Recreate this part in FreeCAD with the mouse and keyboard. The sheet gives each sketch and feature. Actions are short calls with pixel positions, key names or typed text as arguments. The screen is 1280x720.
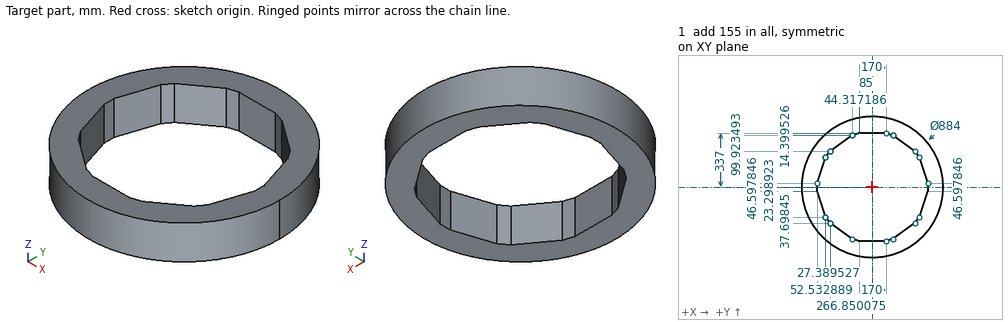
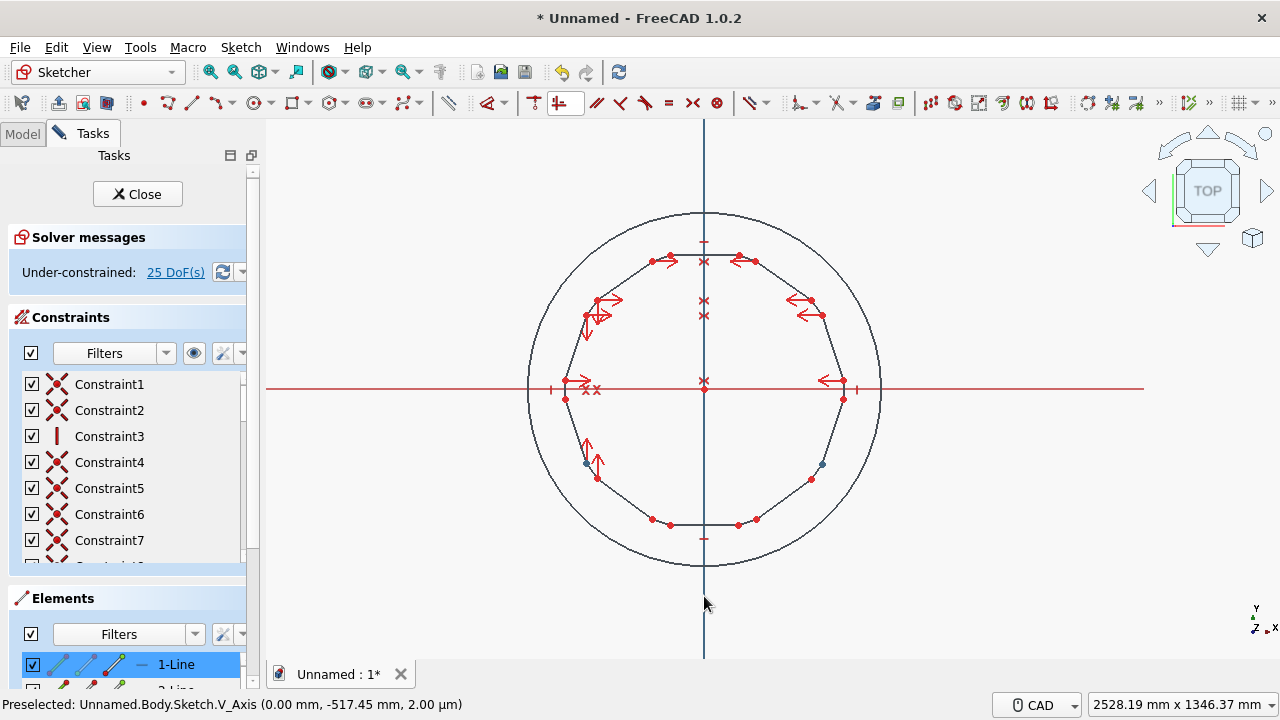
key(s)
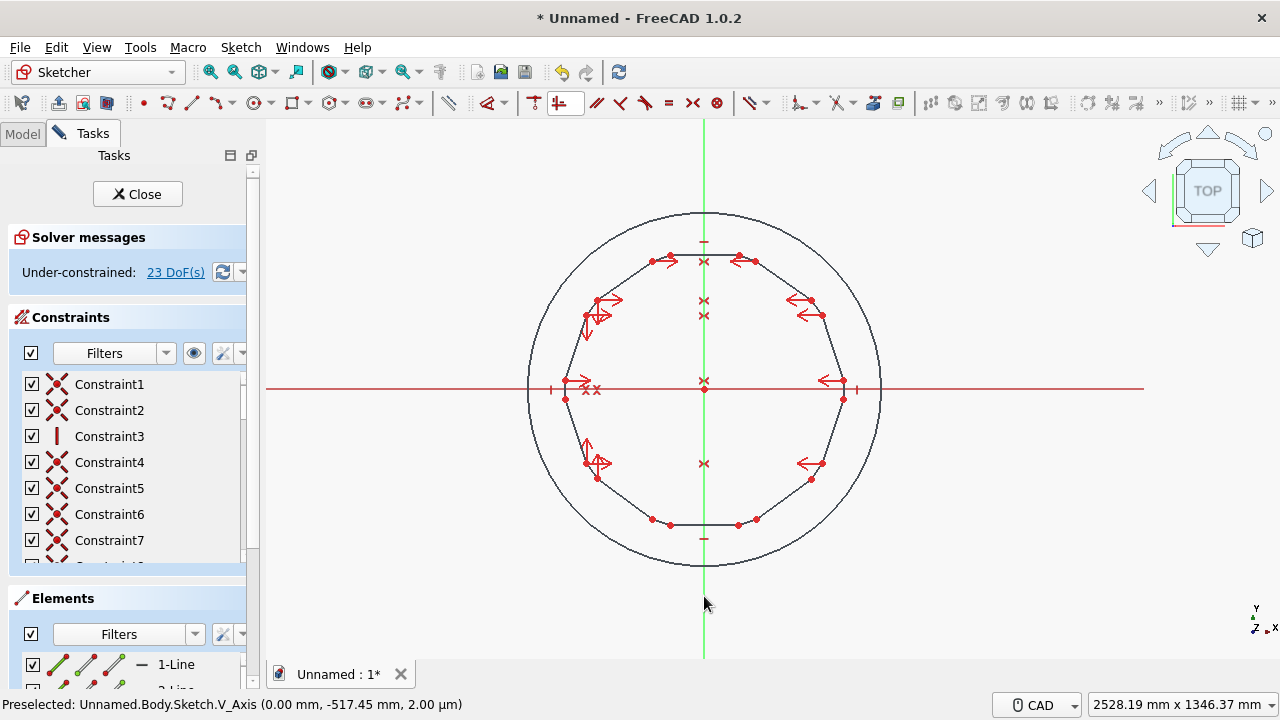
click(598, 479)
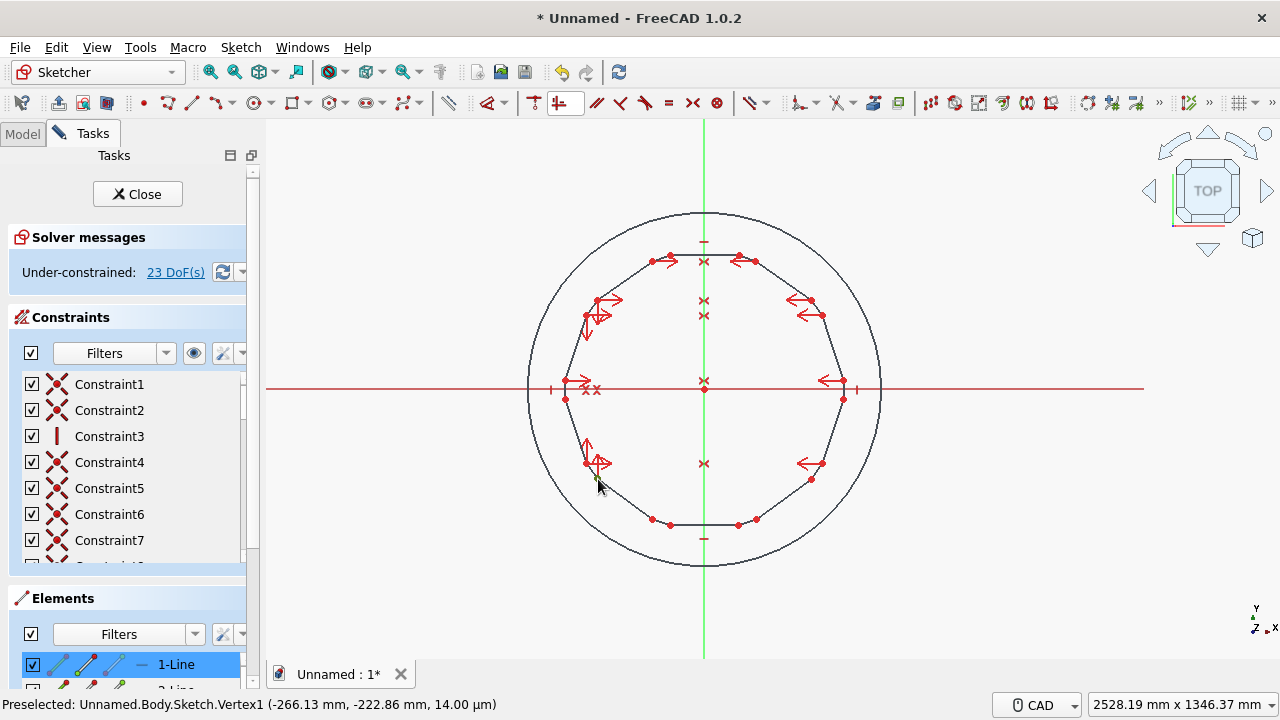
click(811, 479)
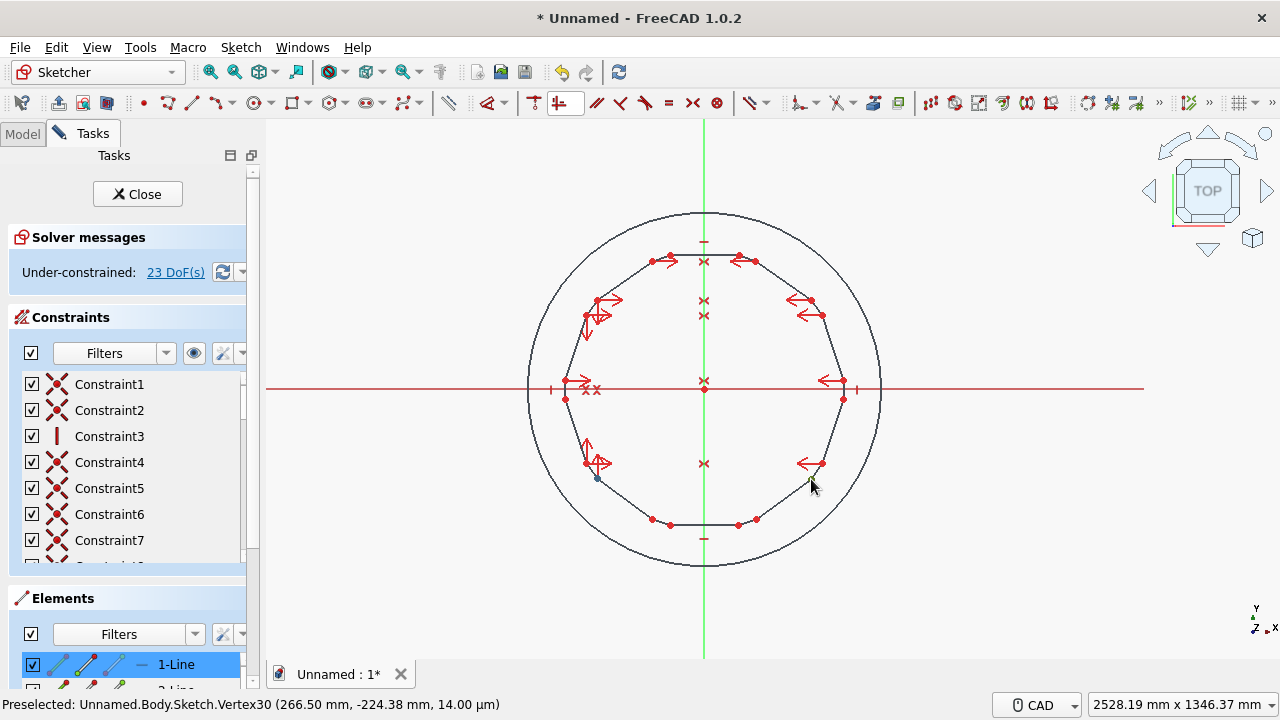
click(704, 596)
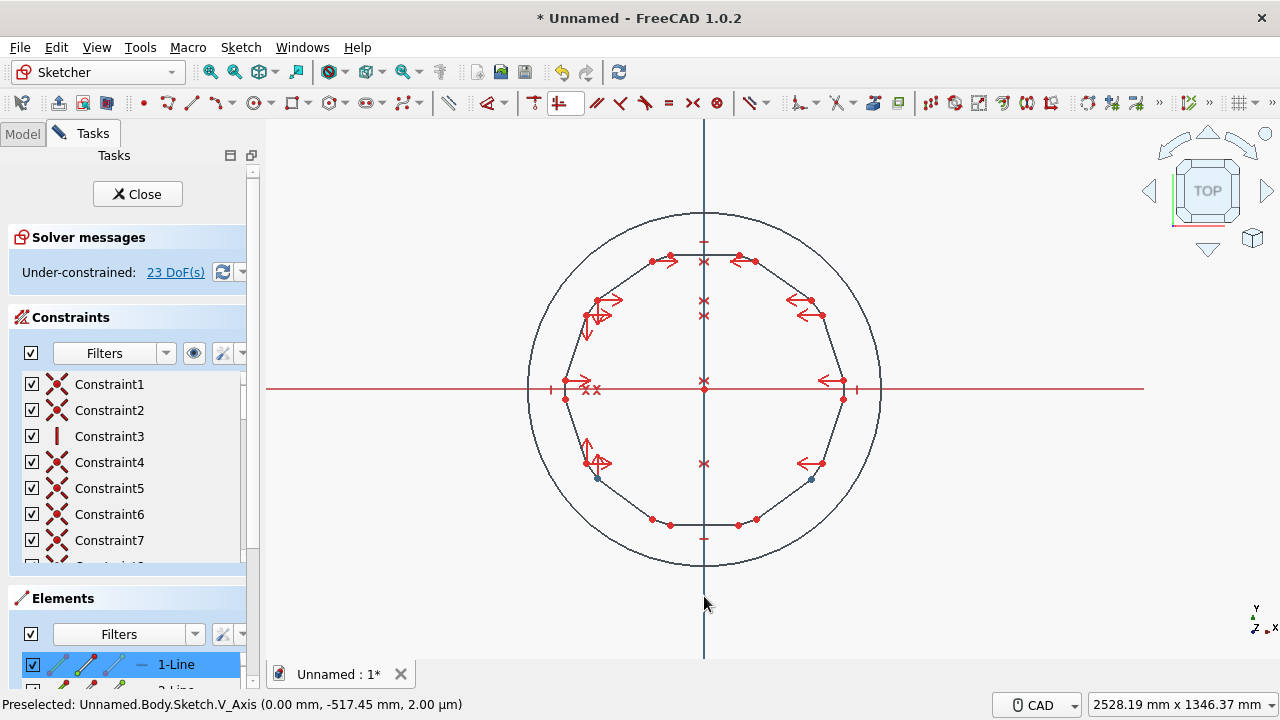
click(694, 104)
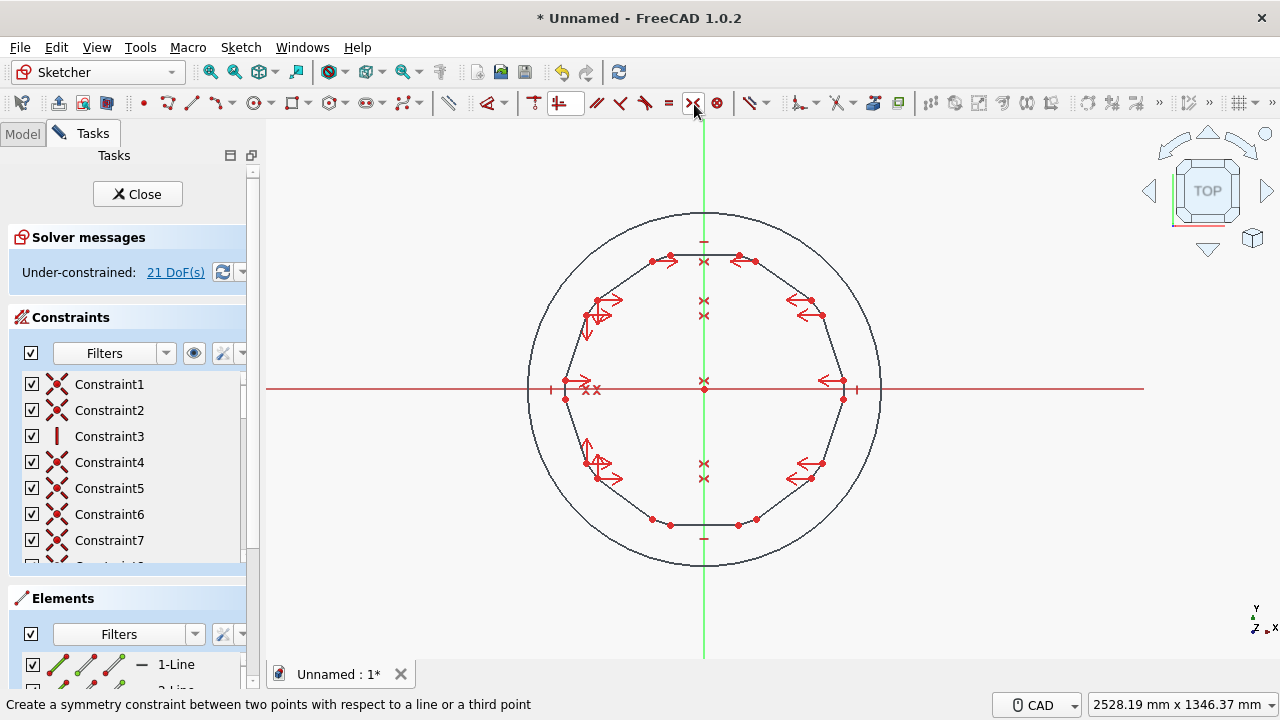
click(756, 261)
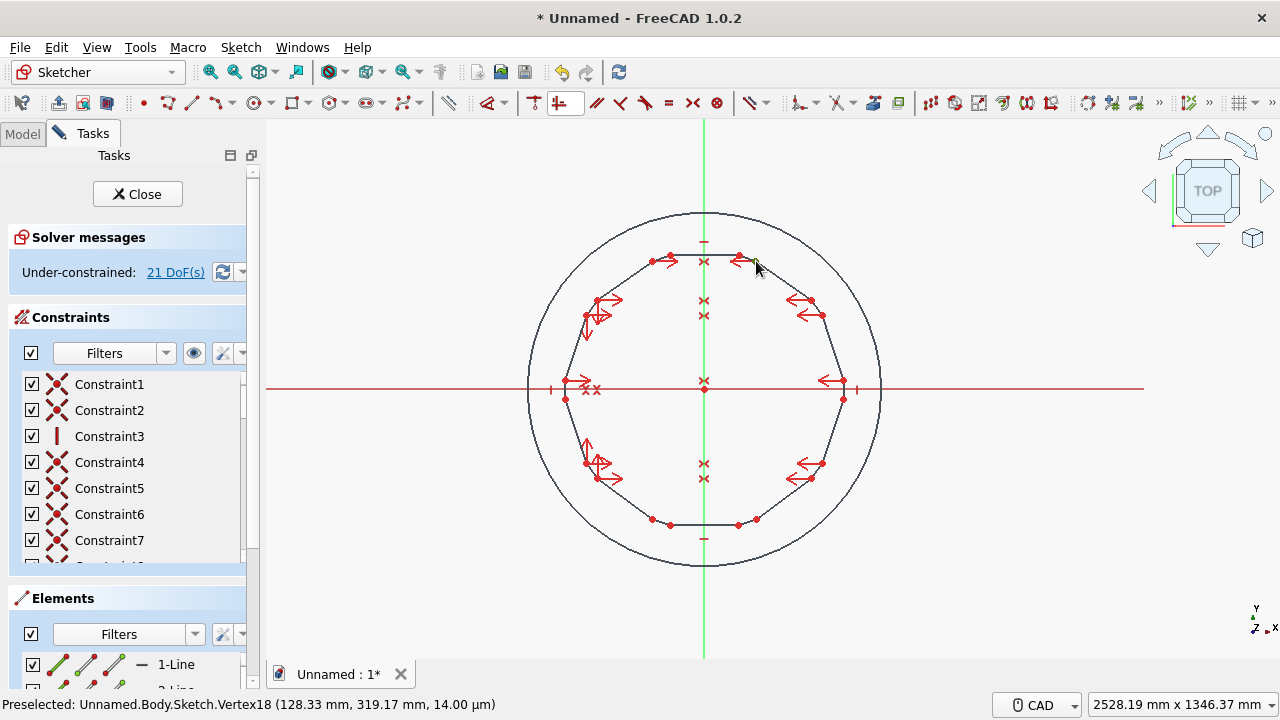
click(757, 519)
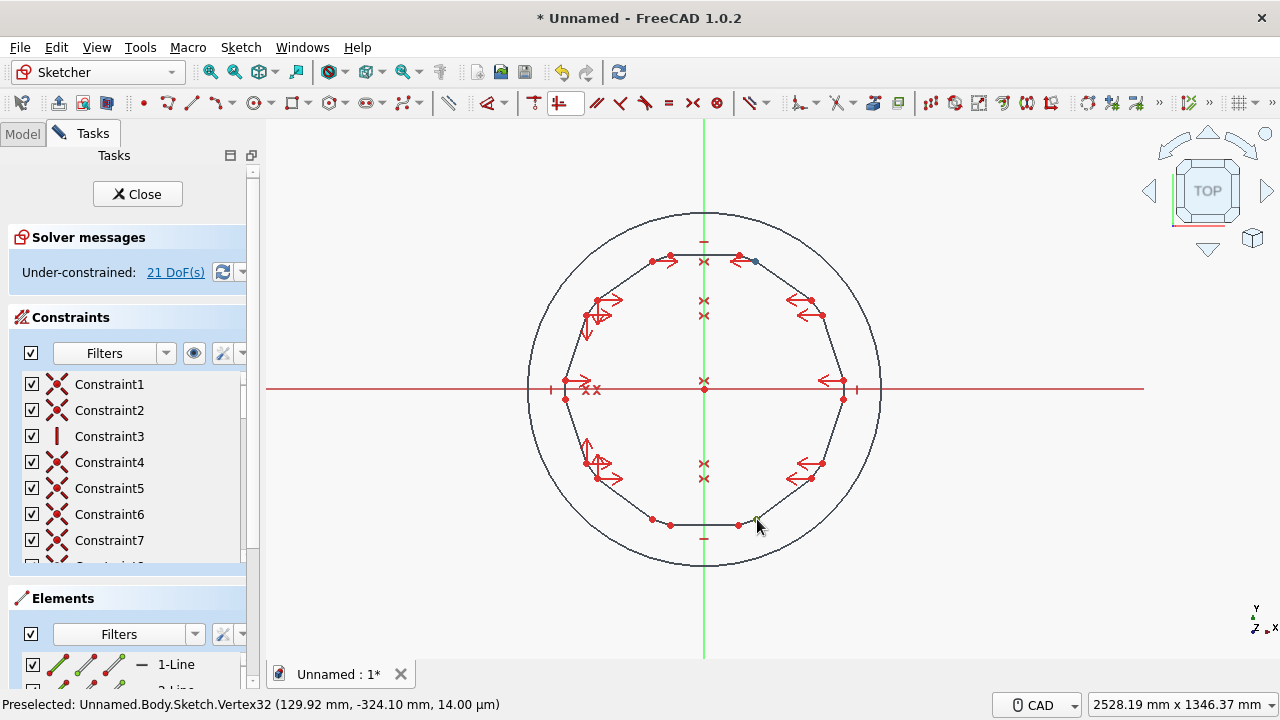
click(353, 389)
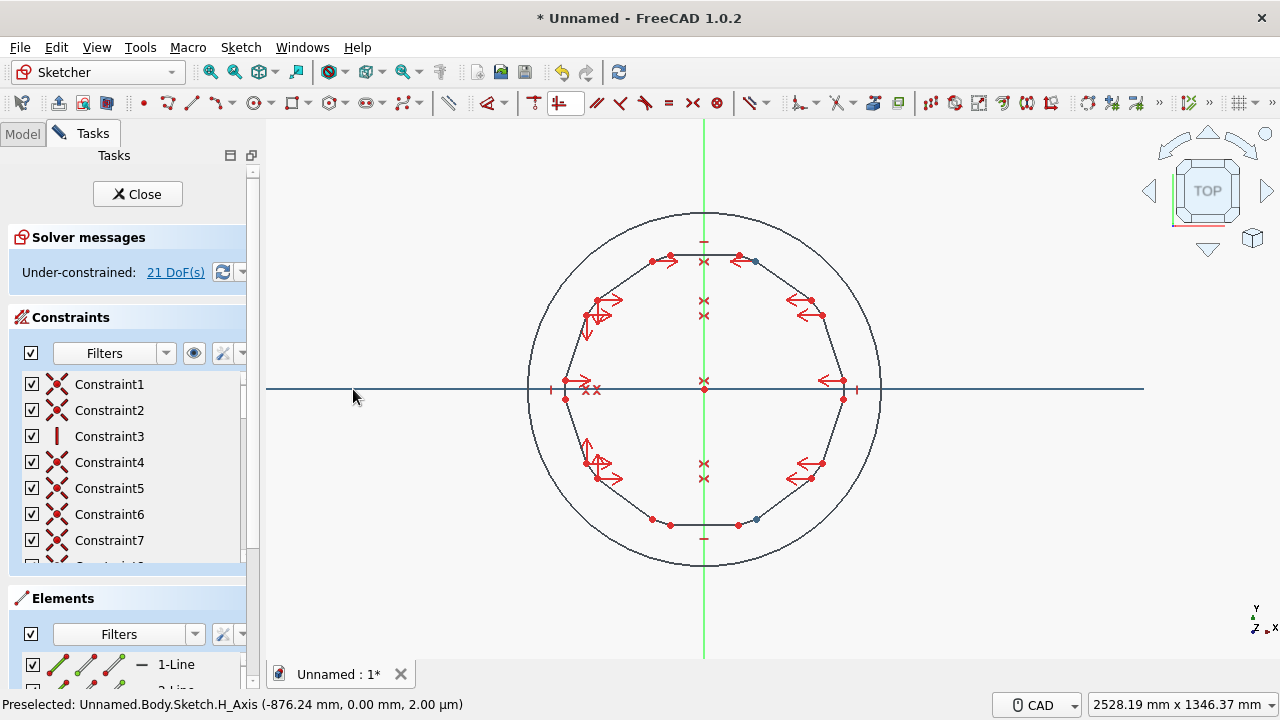
key(s)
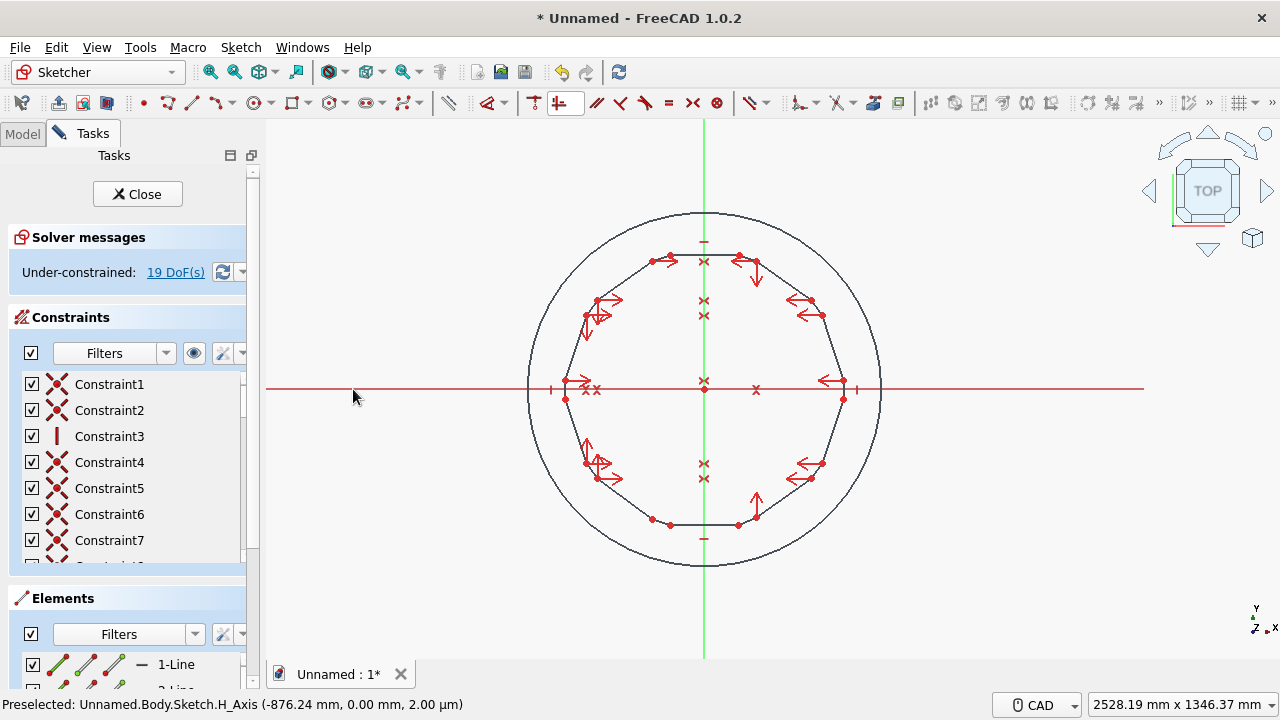
click(739, 255)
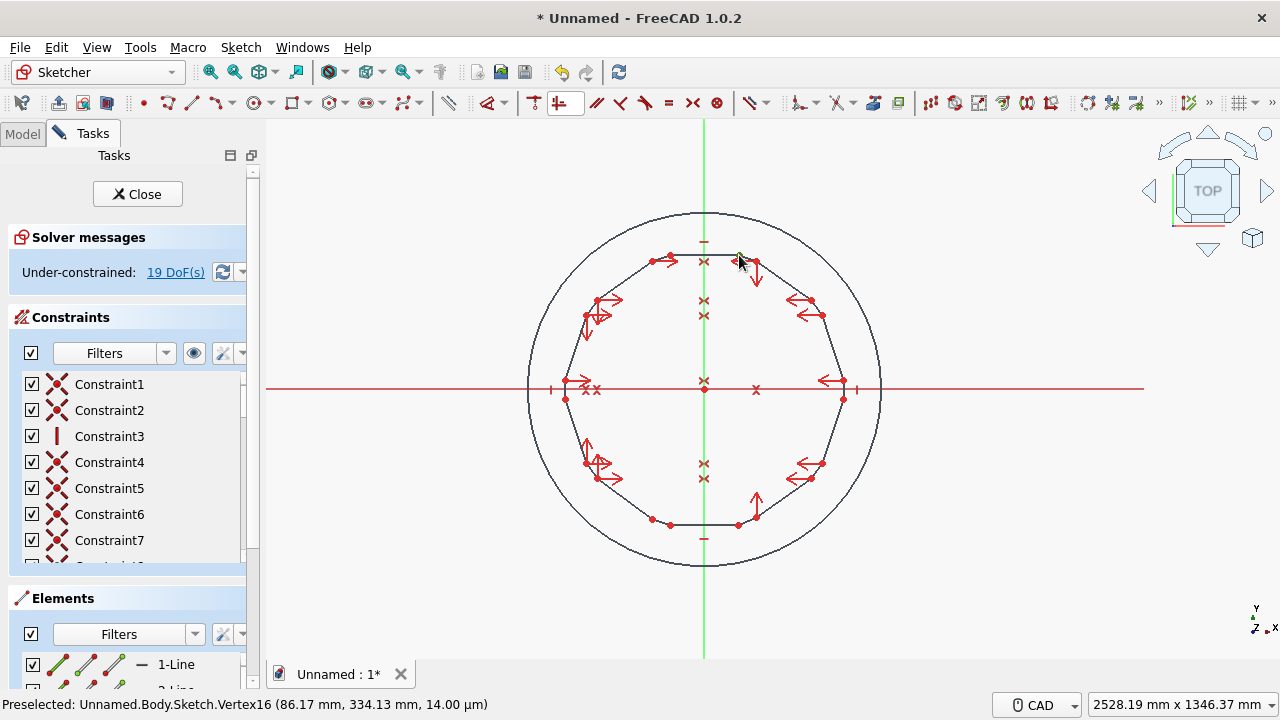
click(739, 525)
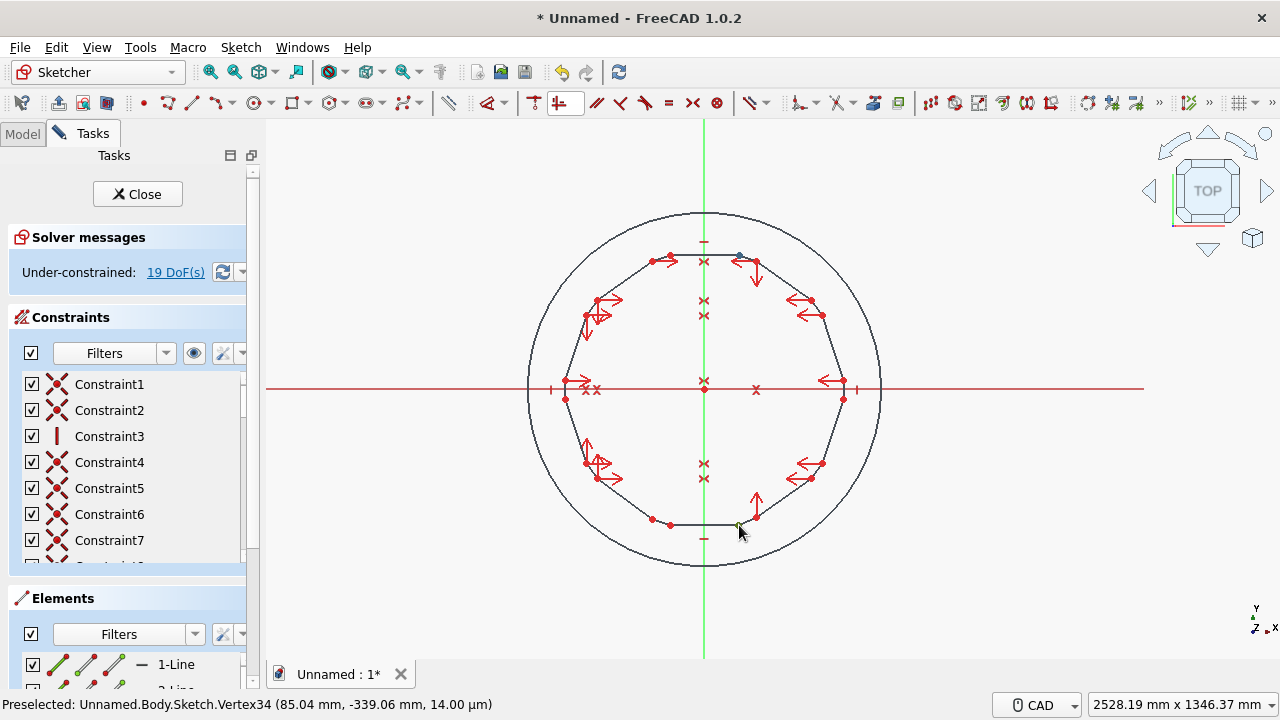
click(353, 389)